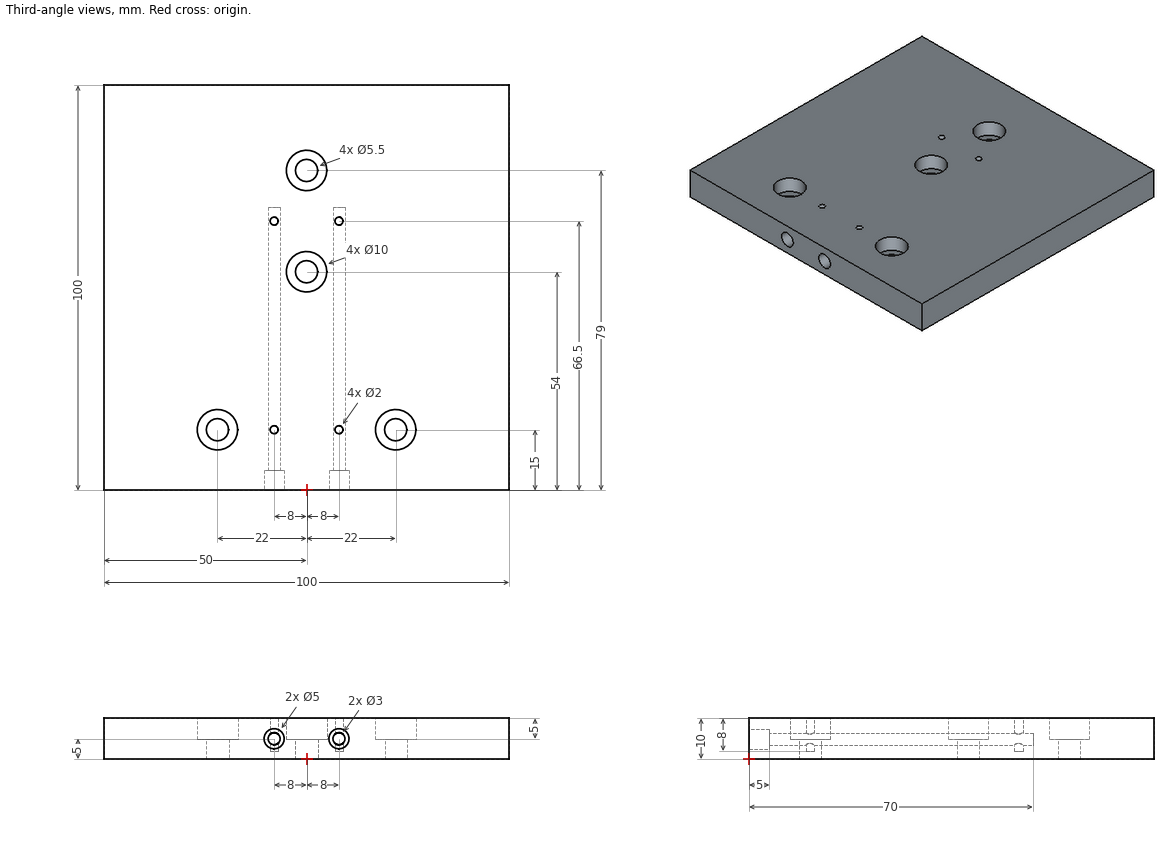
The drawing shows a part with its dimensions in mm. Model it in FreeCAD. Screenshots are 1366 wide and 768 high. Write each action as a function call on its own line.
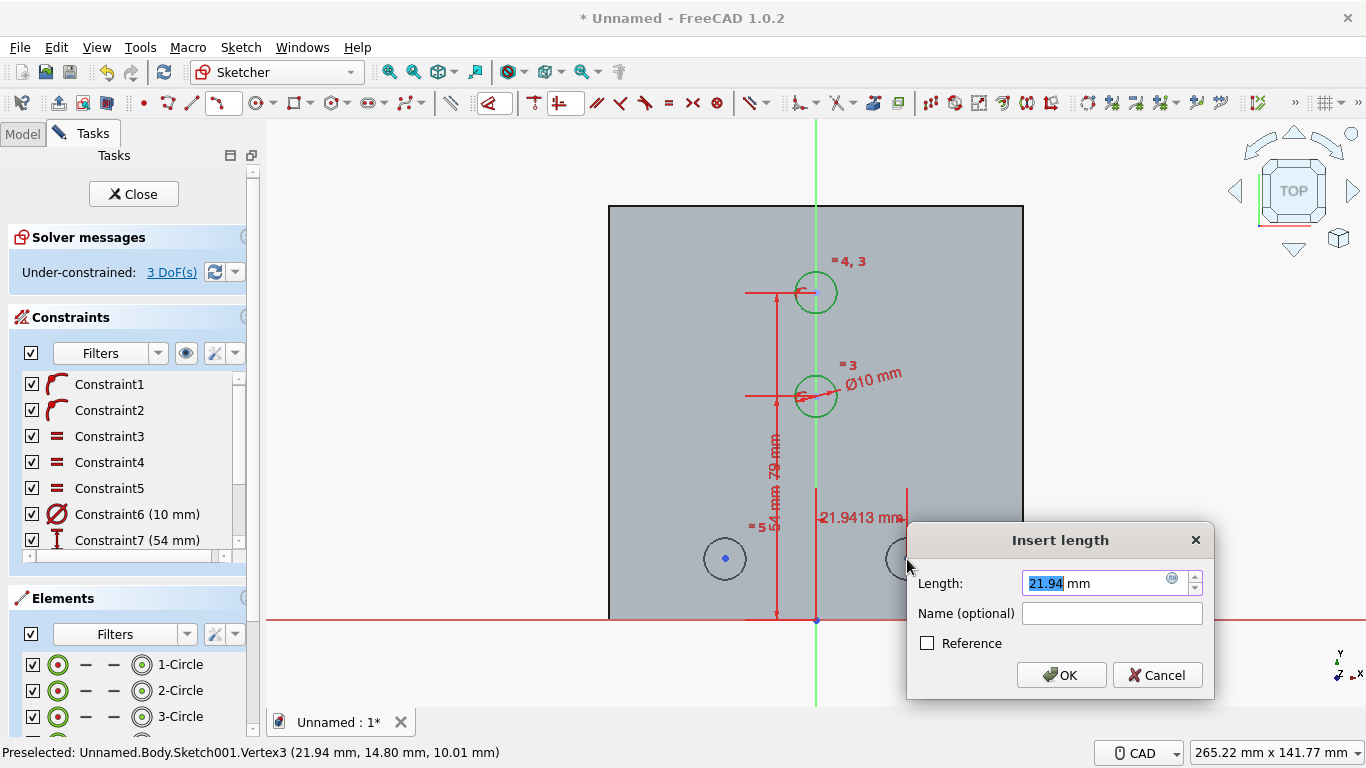
text(22)
key(Return)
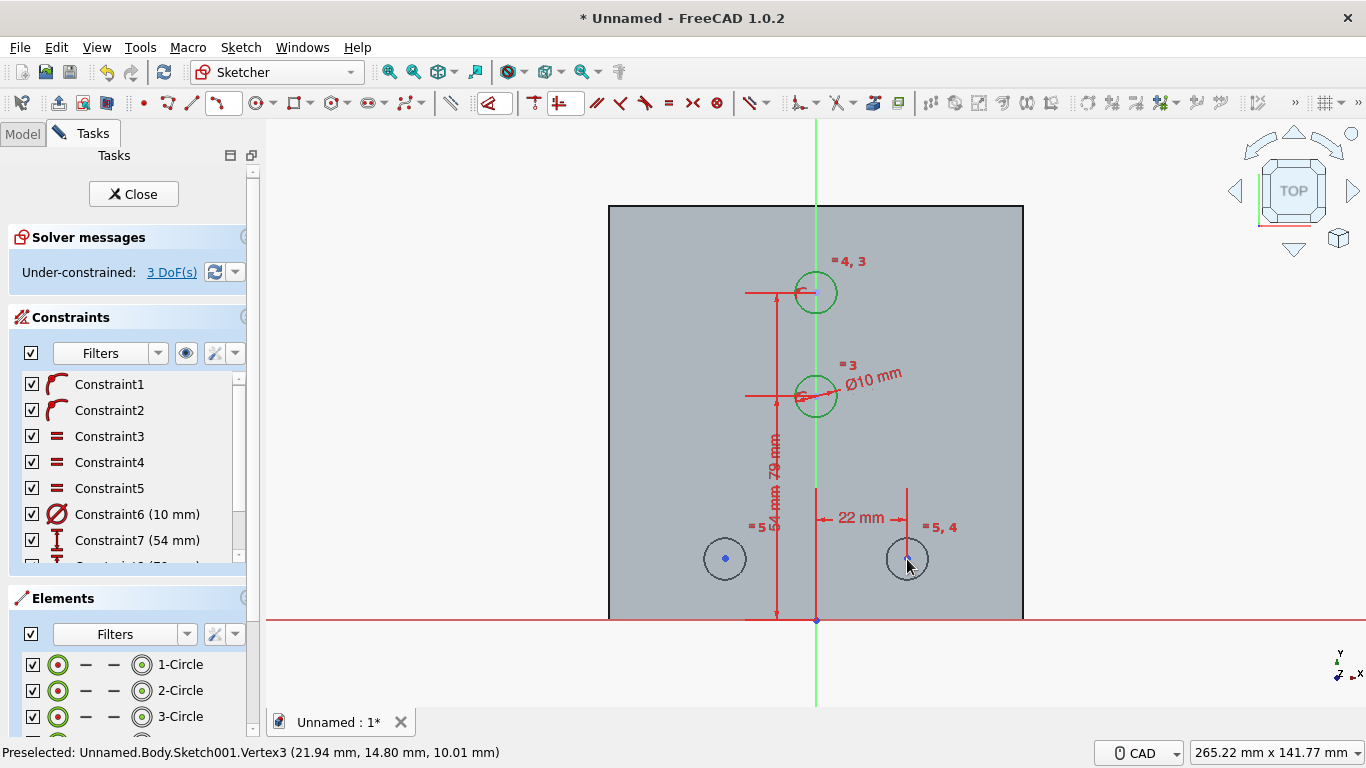
click(907, 559)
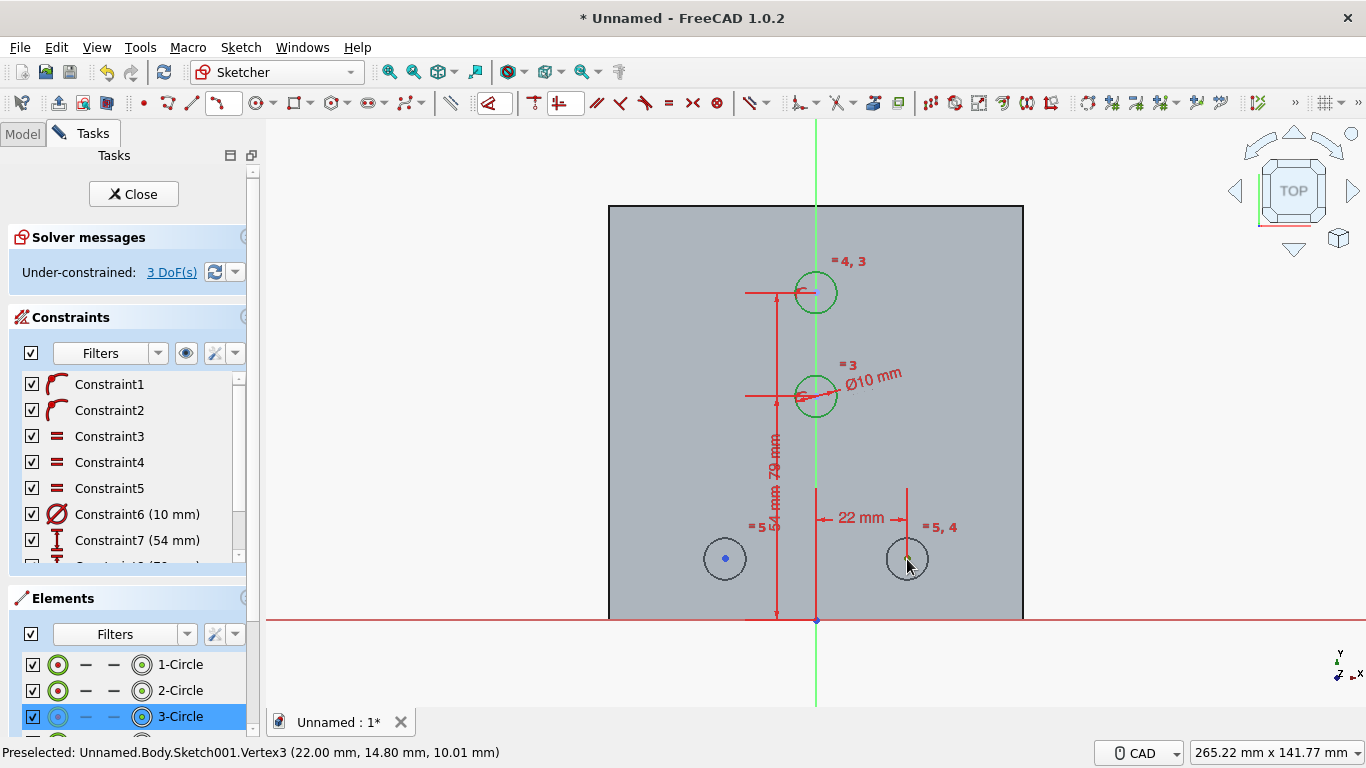
key(i)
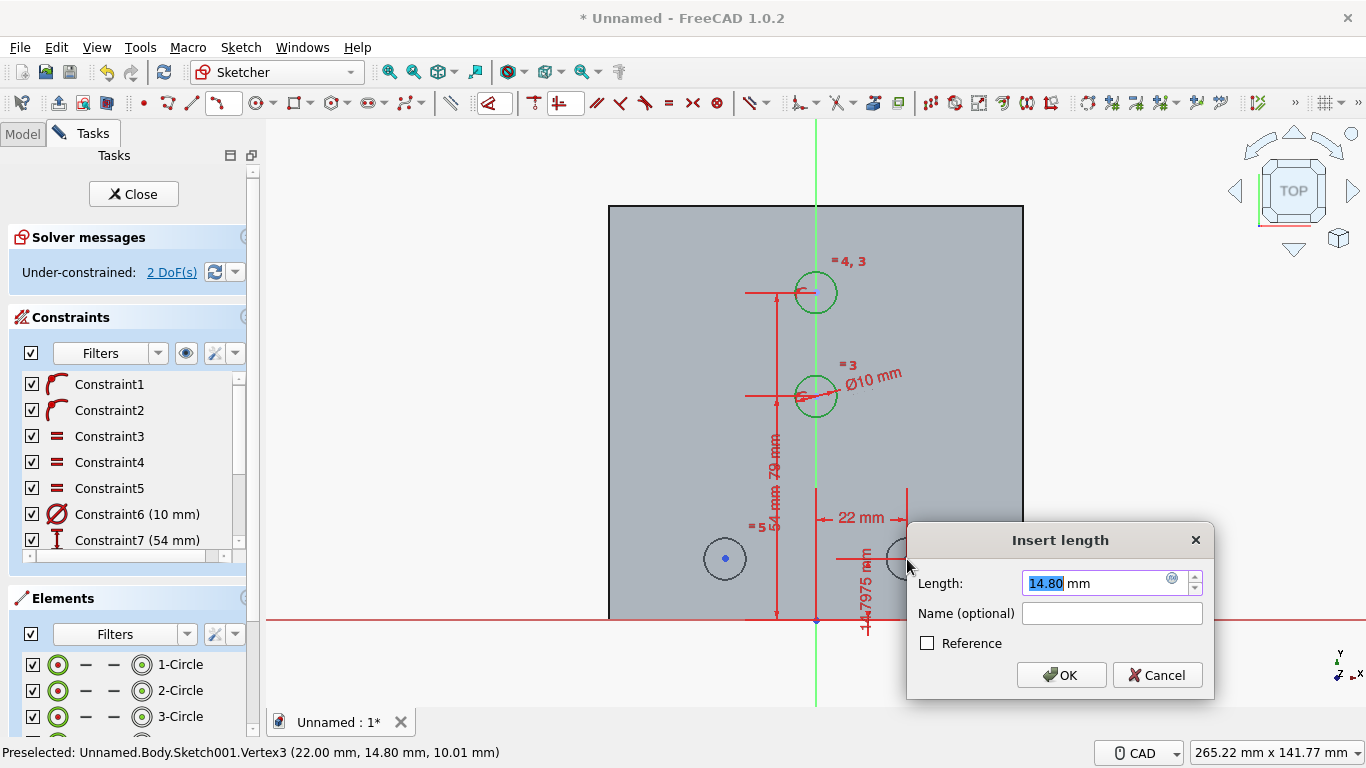
text(15)
key(Return)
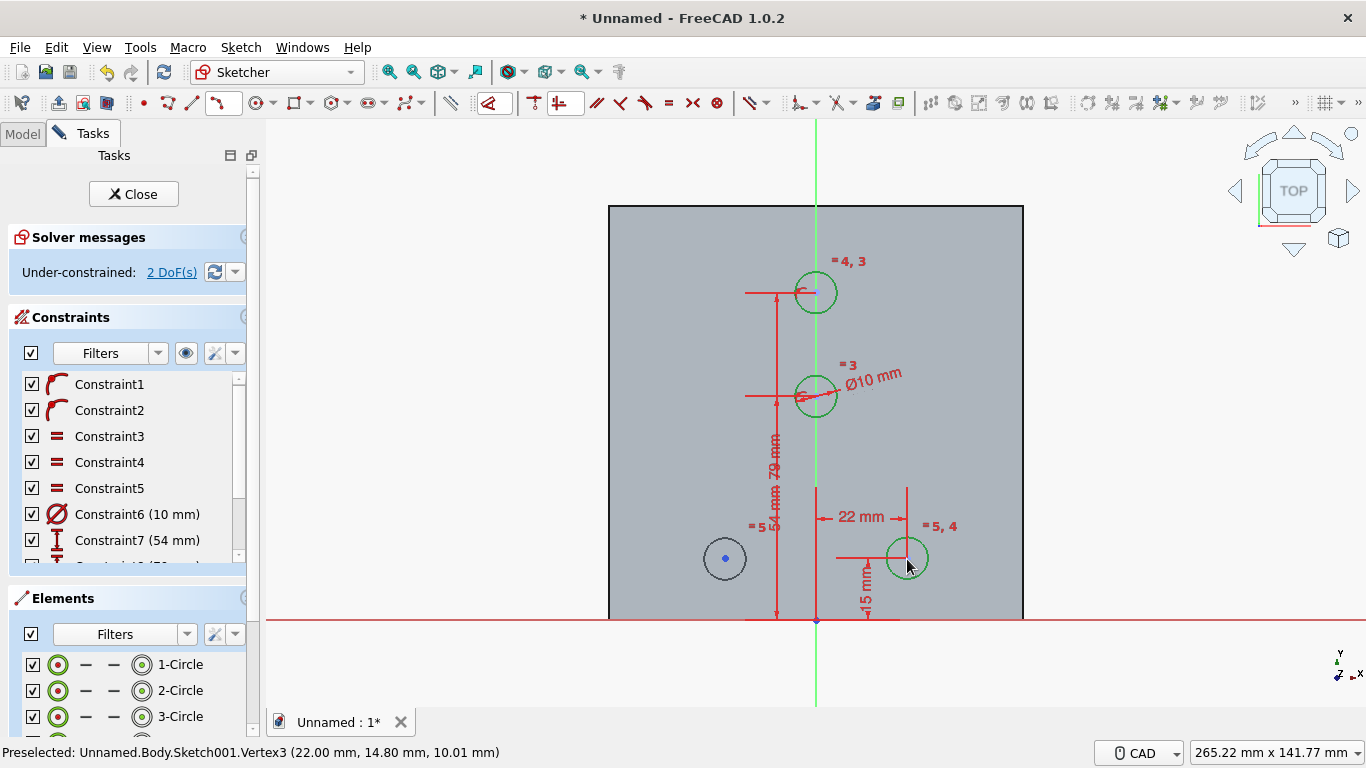
click(725, 559)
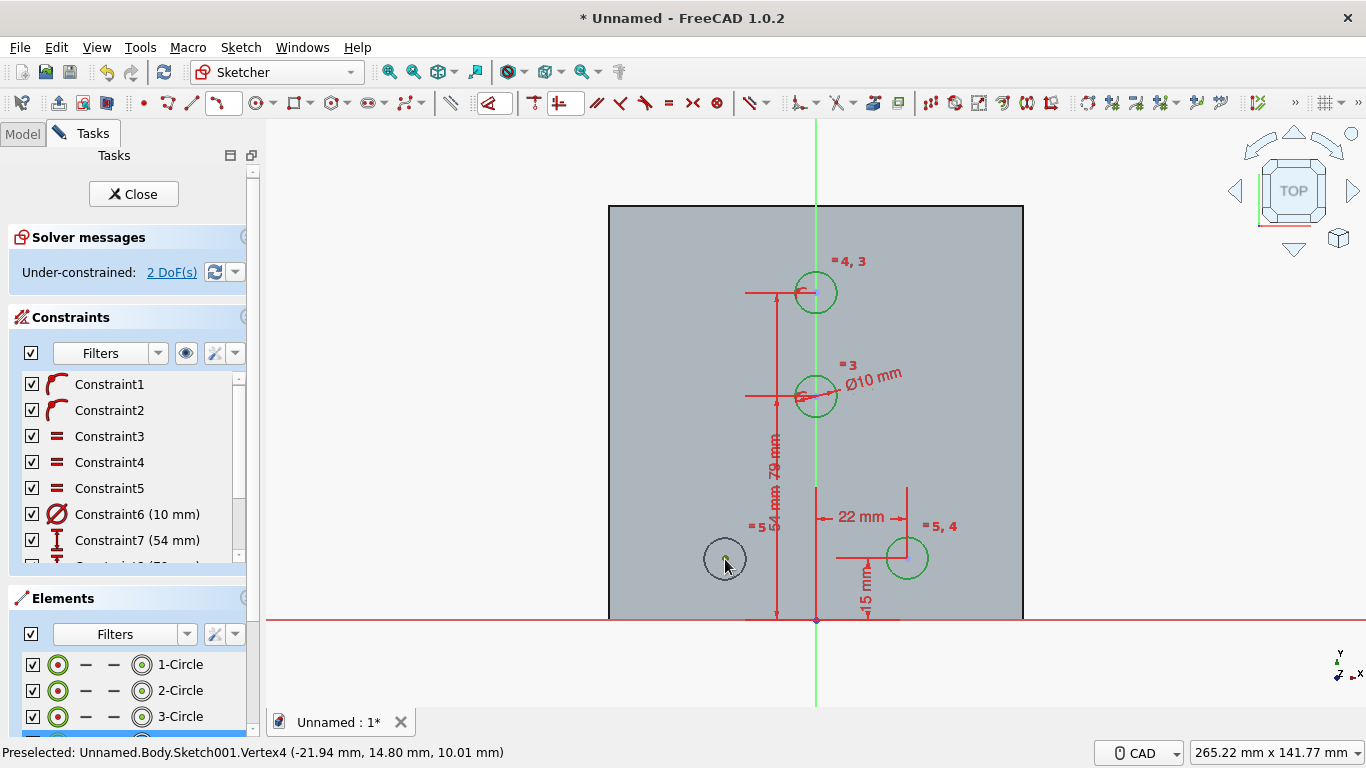
click(506, 104)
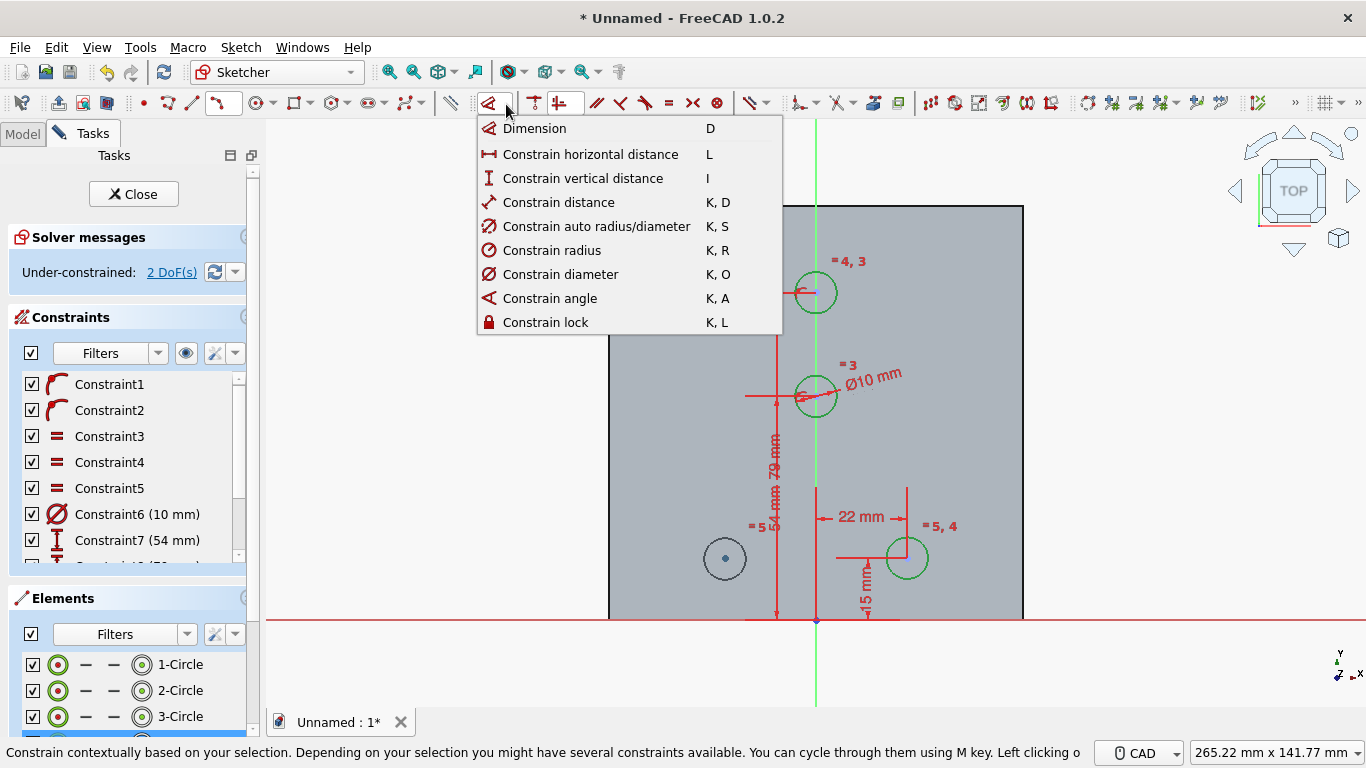
click(630, 154)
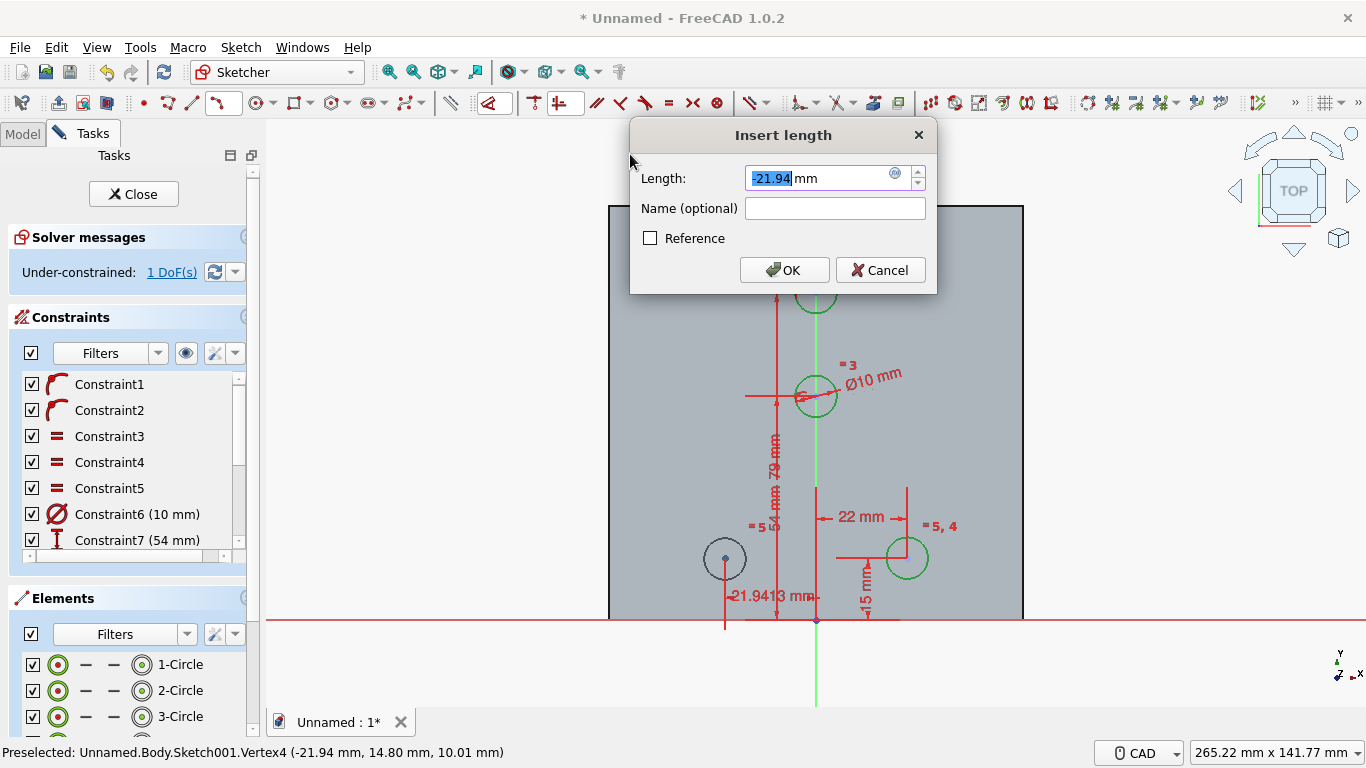
text(-22)
key(Return)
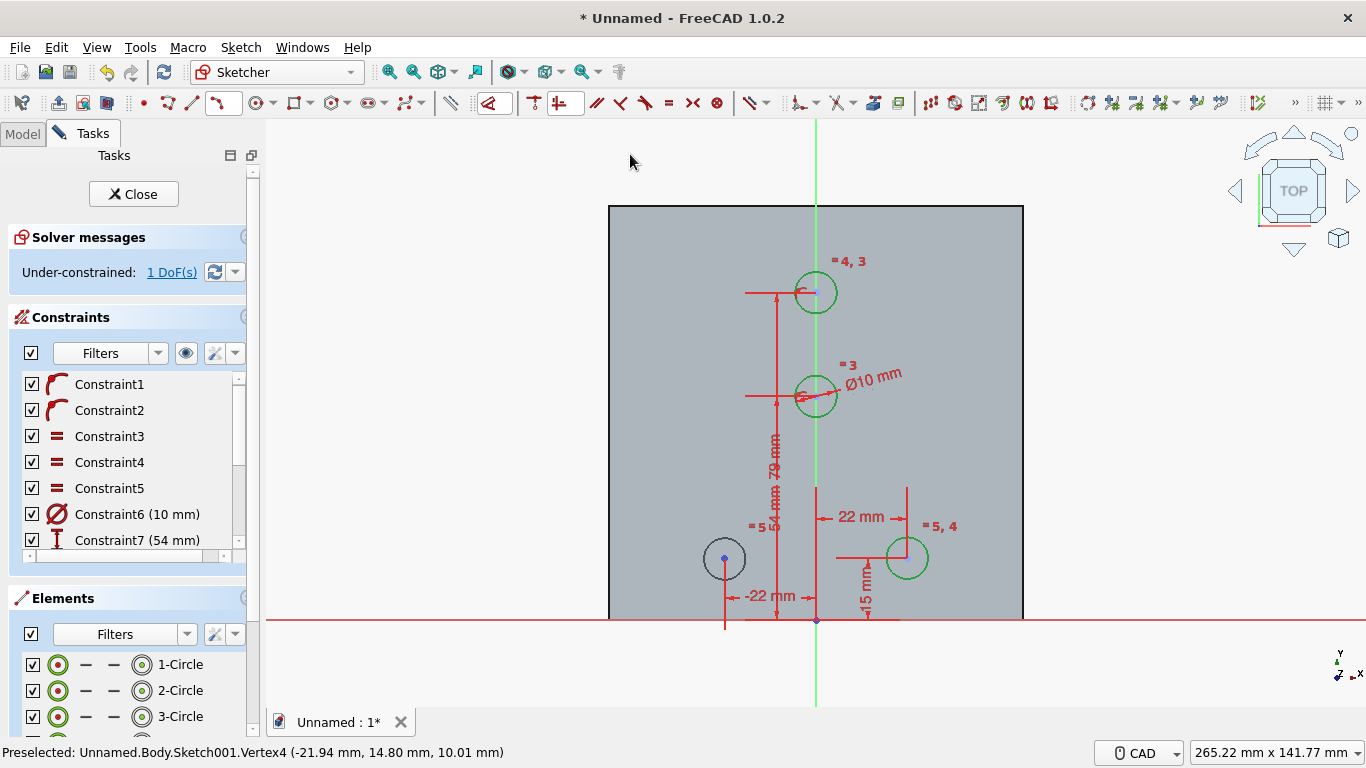
click(725, 559)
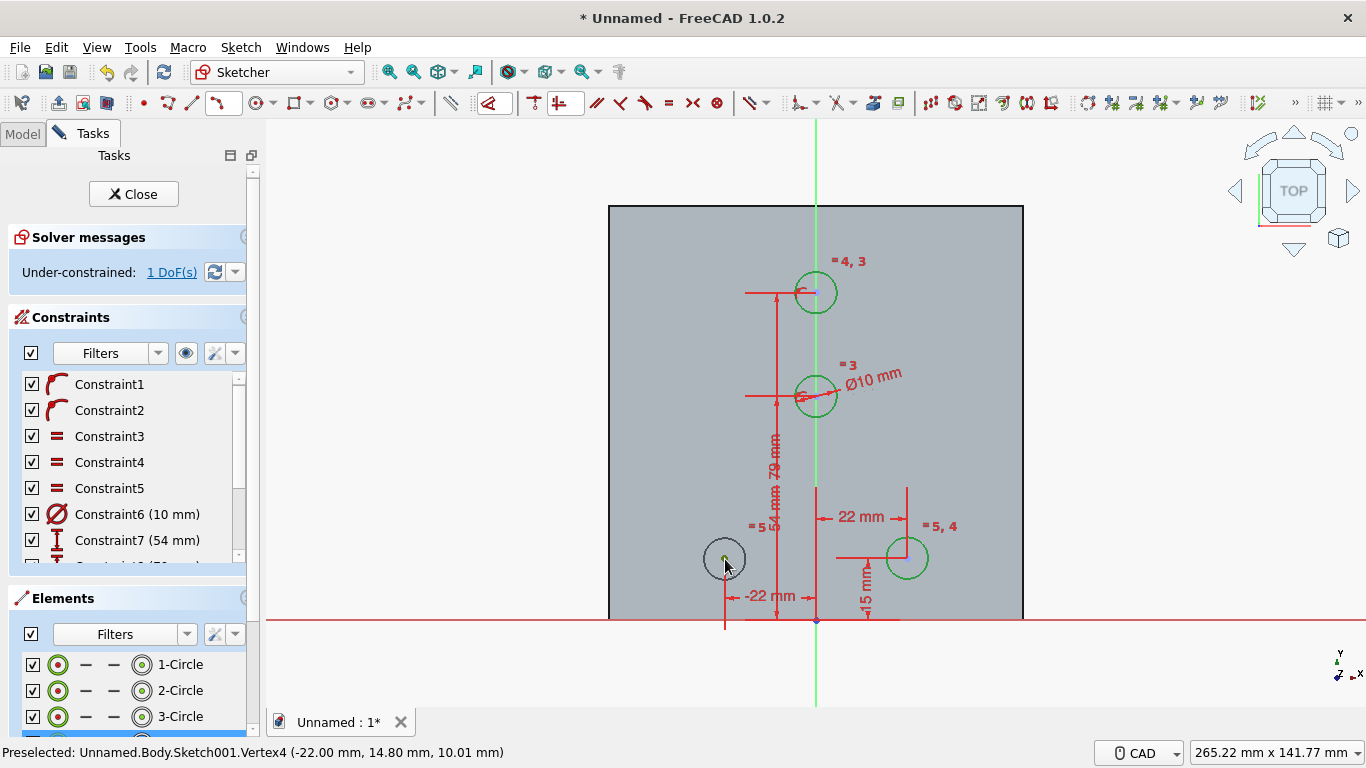
click(506, 104)